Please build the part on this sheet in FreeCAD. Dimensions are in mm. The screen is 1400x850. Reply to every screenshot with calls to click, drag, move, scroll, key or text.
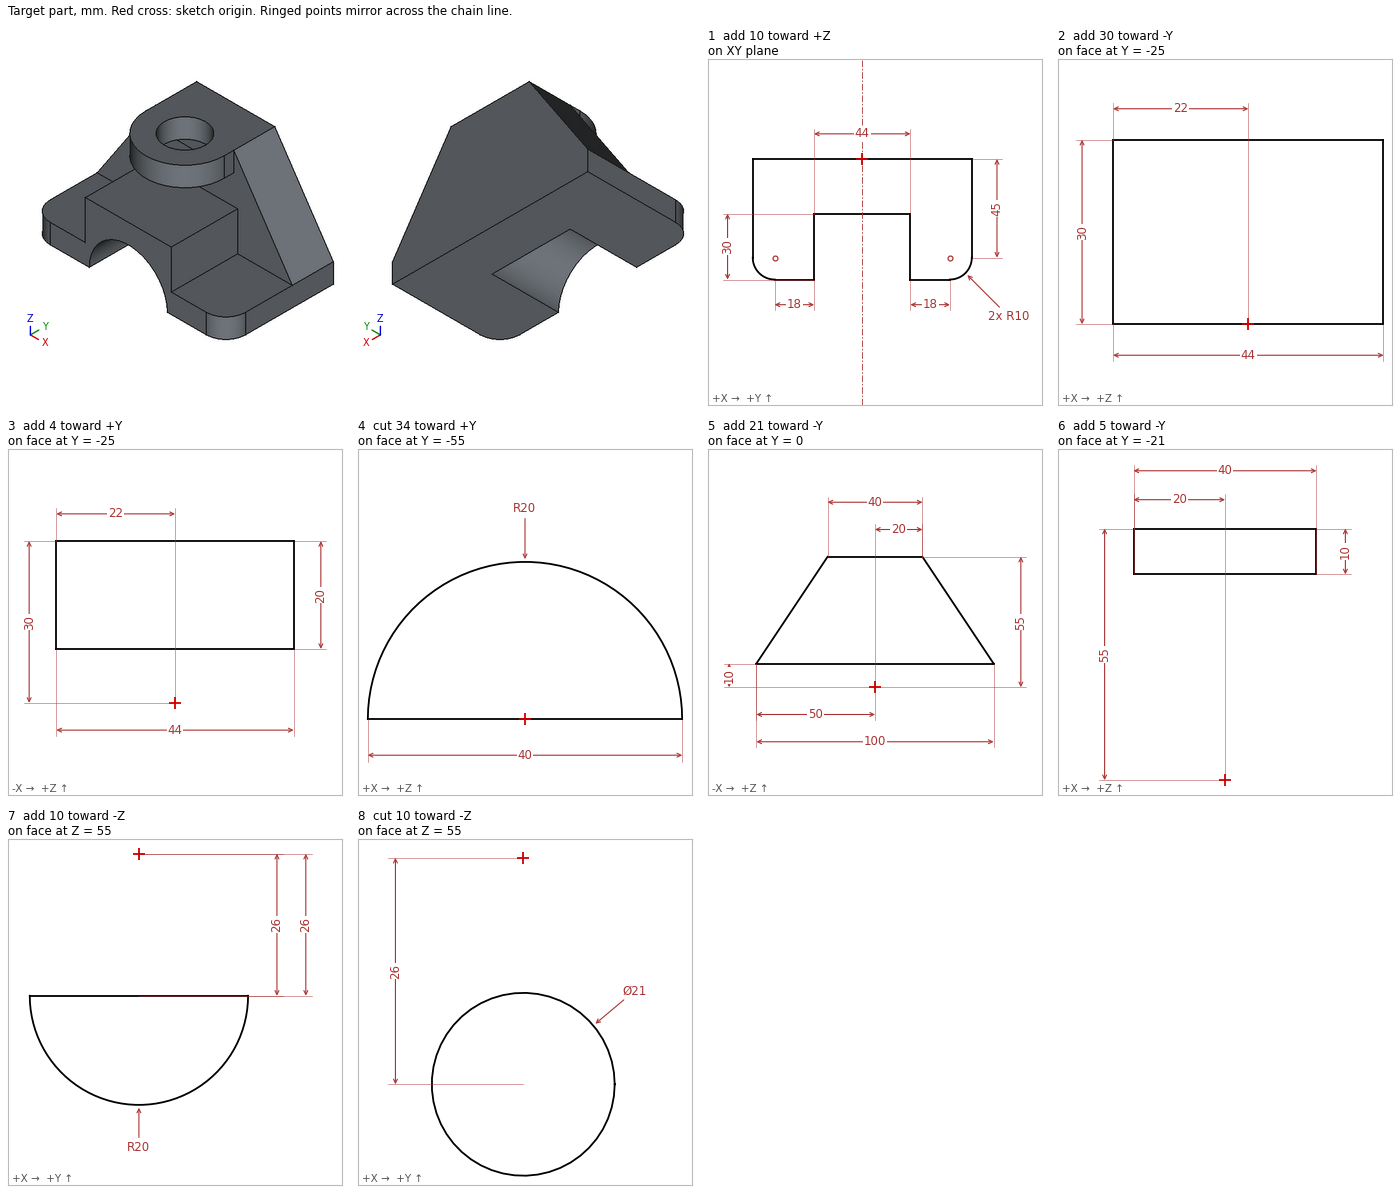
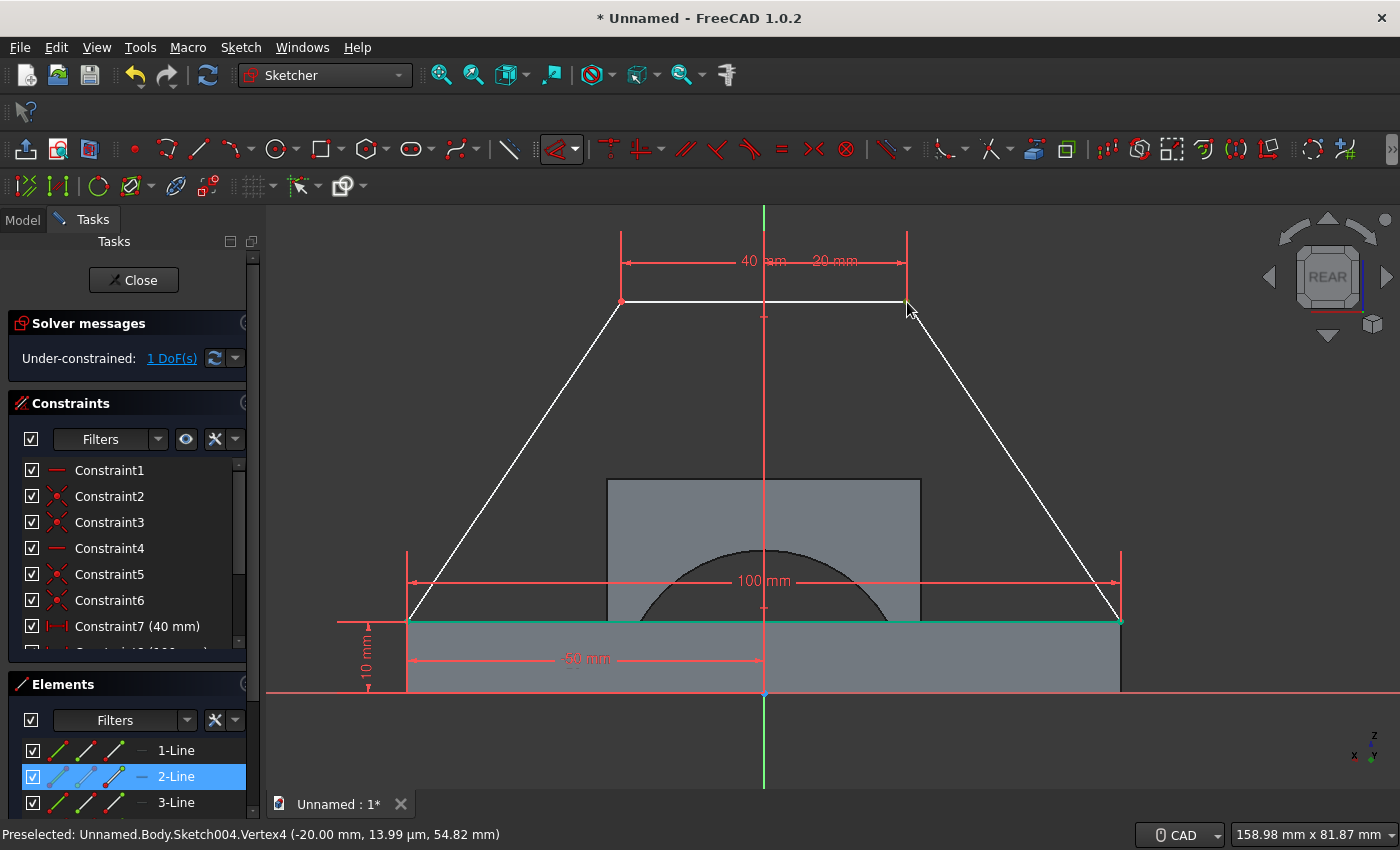
click(578, 150)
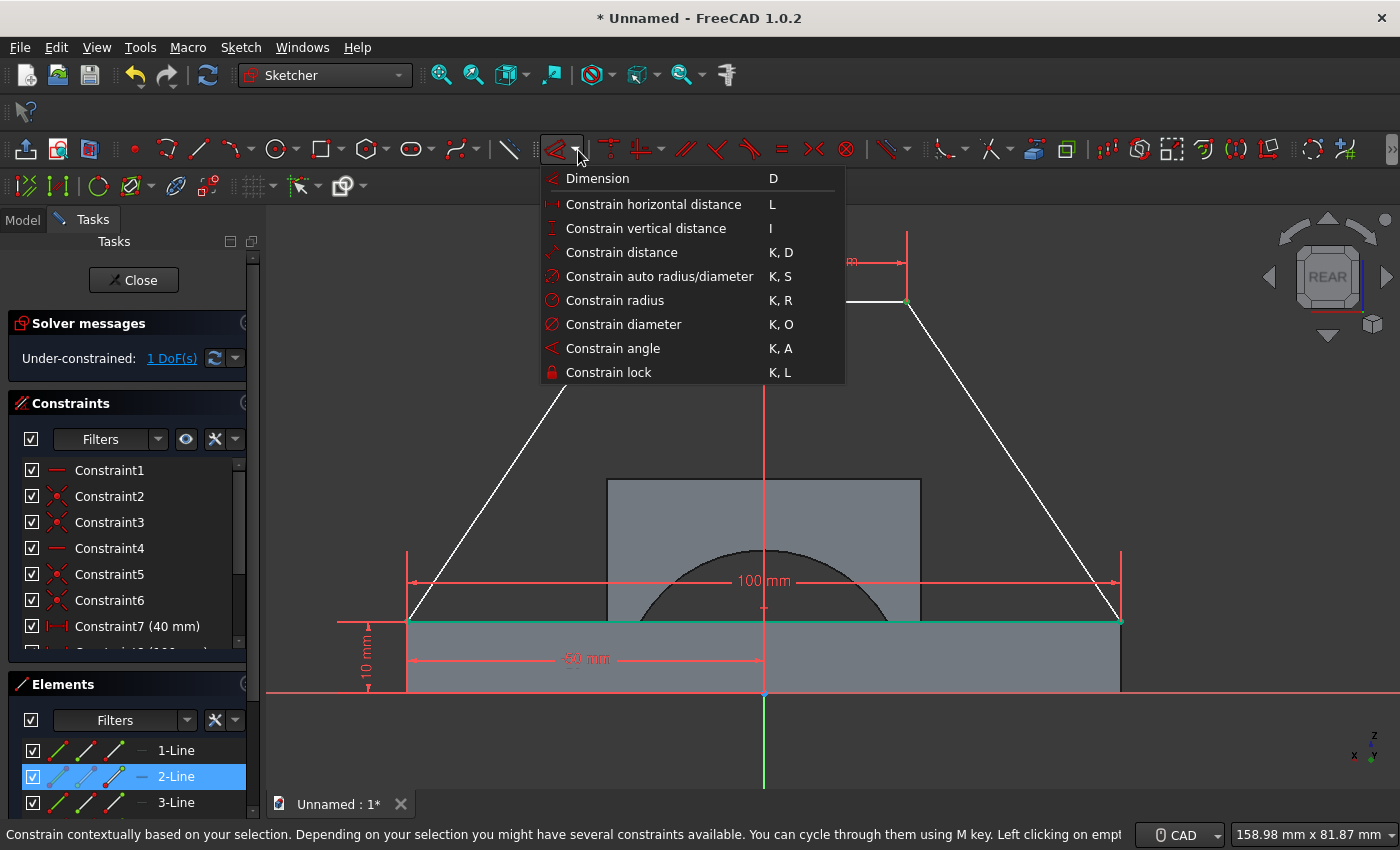
click(693, 228)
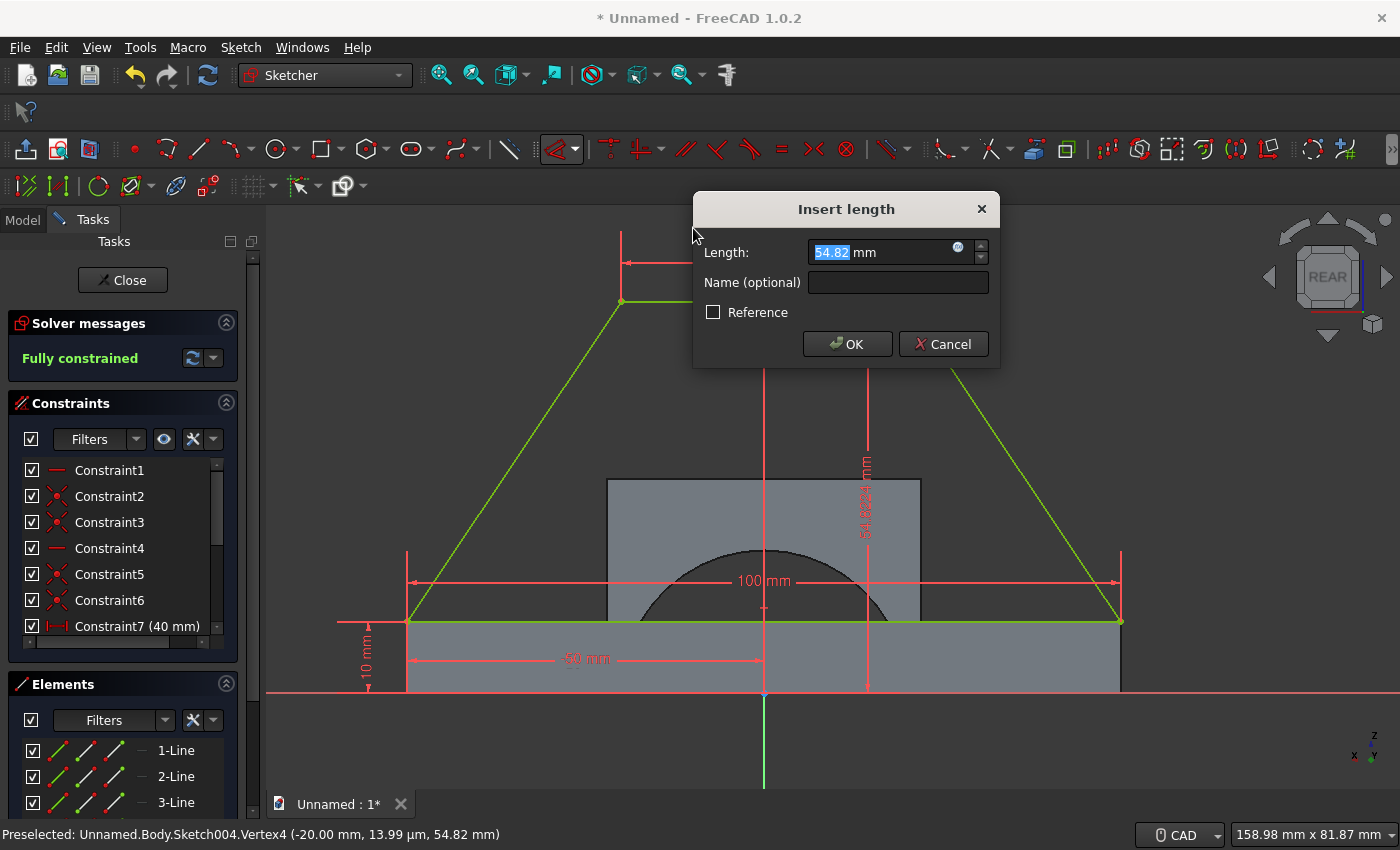
text(55)
key(Return)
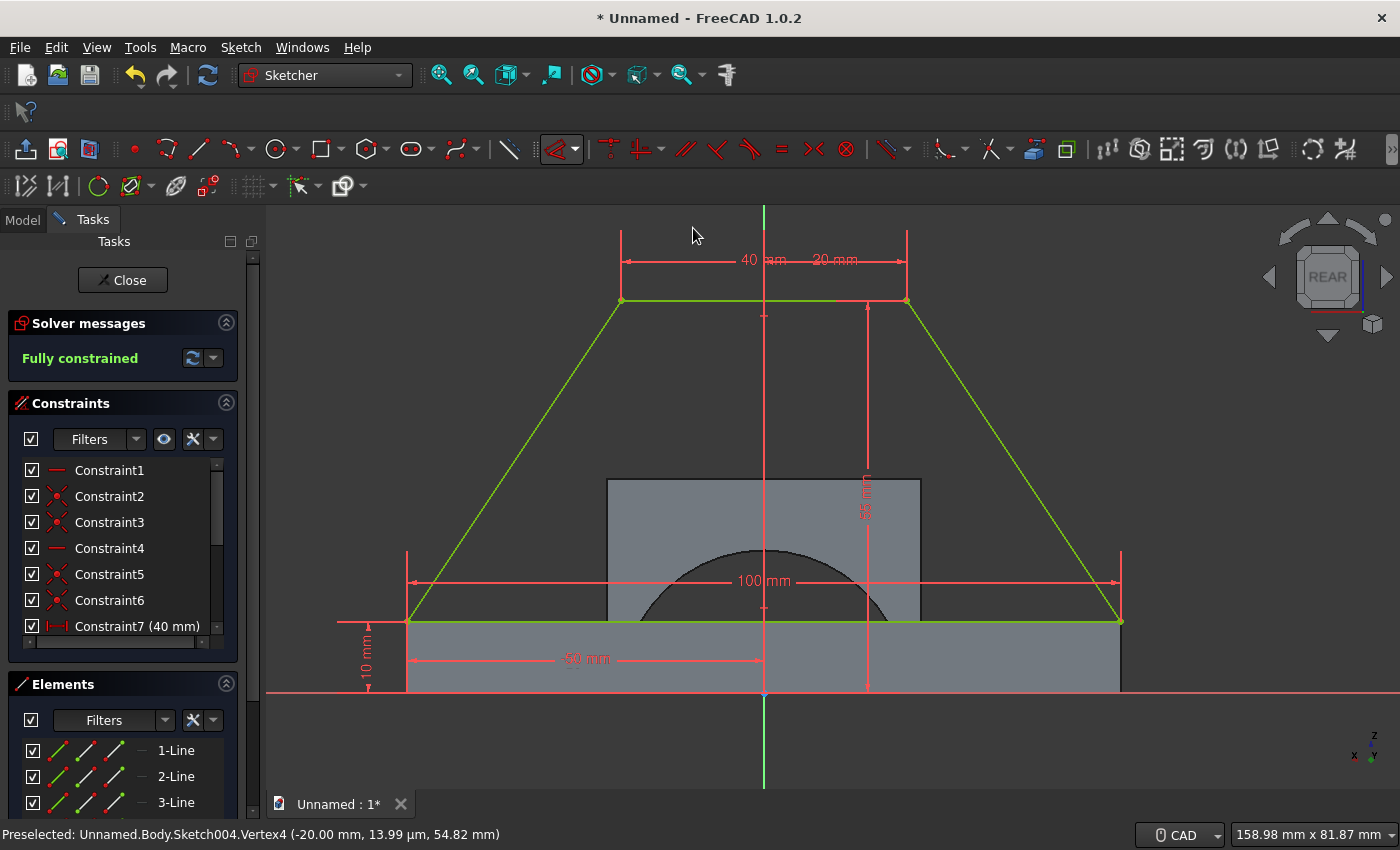
click(123, 280)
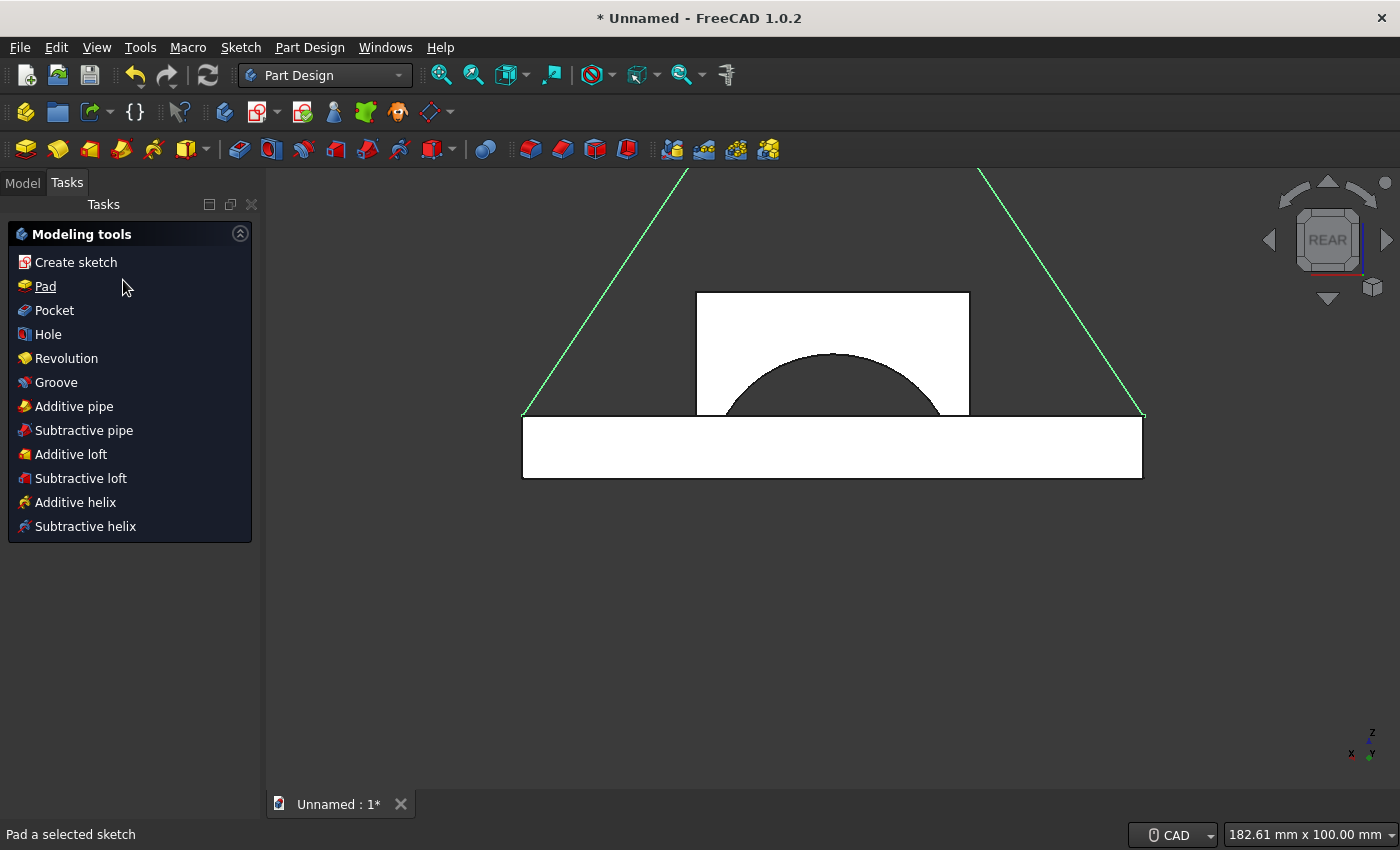
click(26, 150)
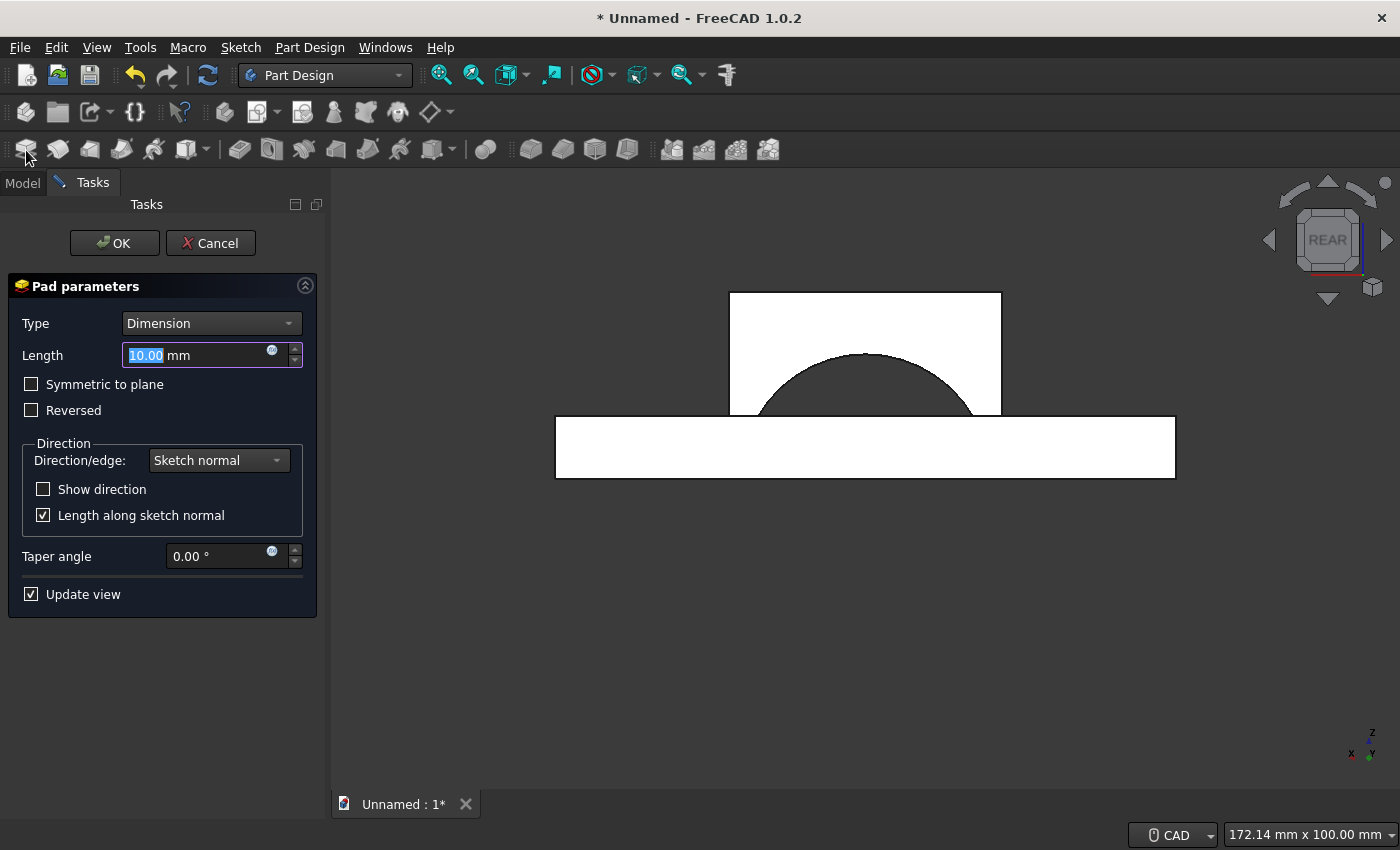
text(21)
key(Tab)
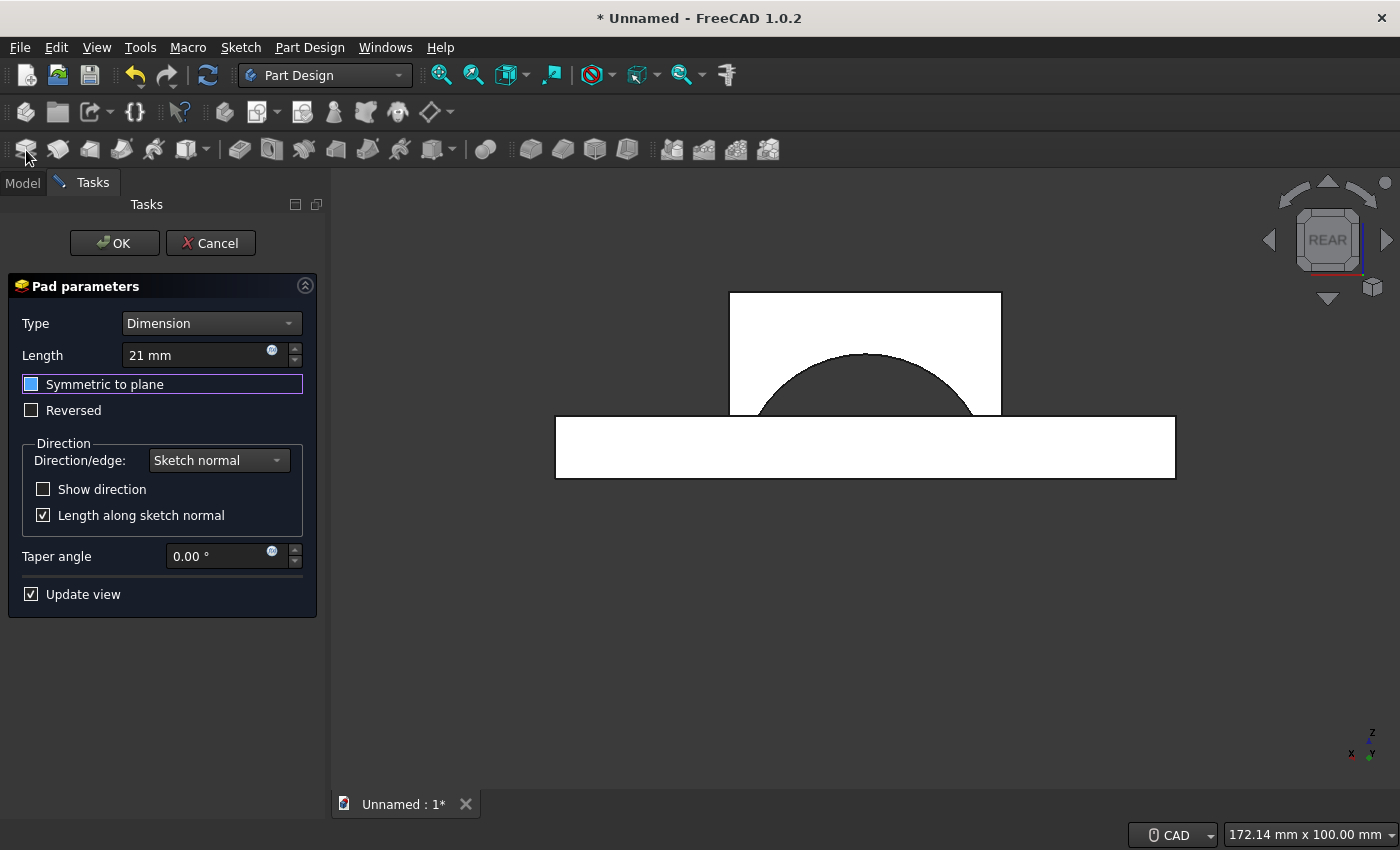
click(30, 410)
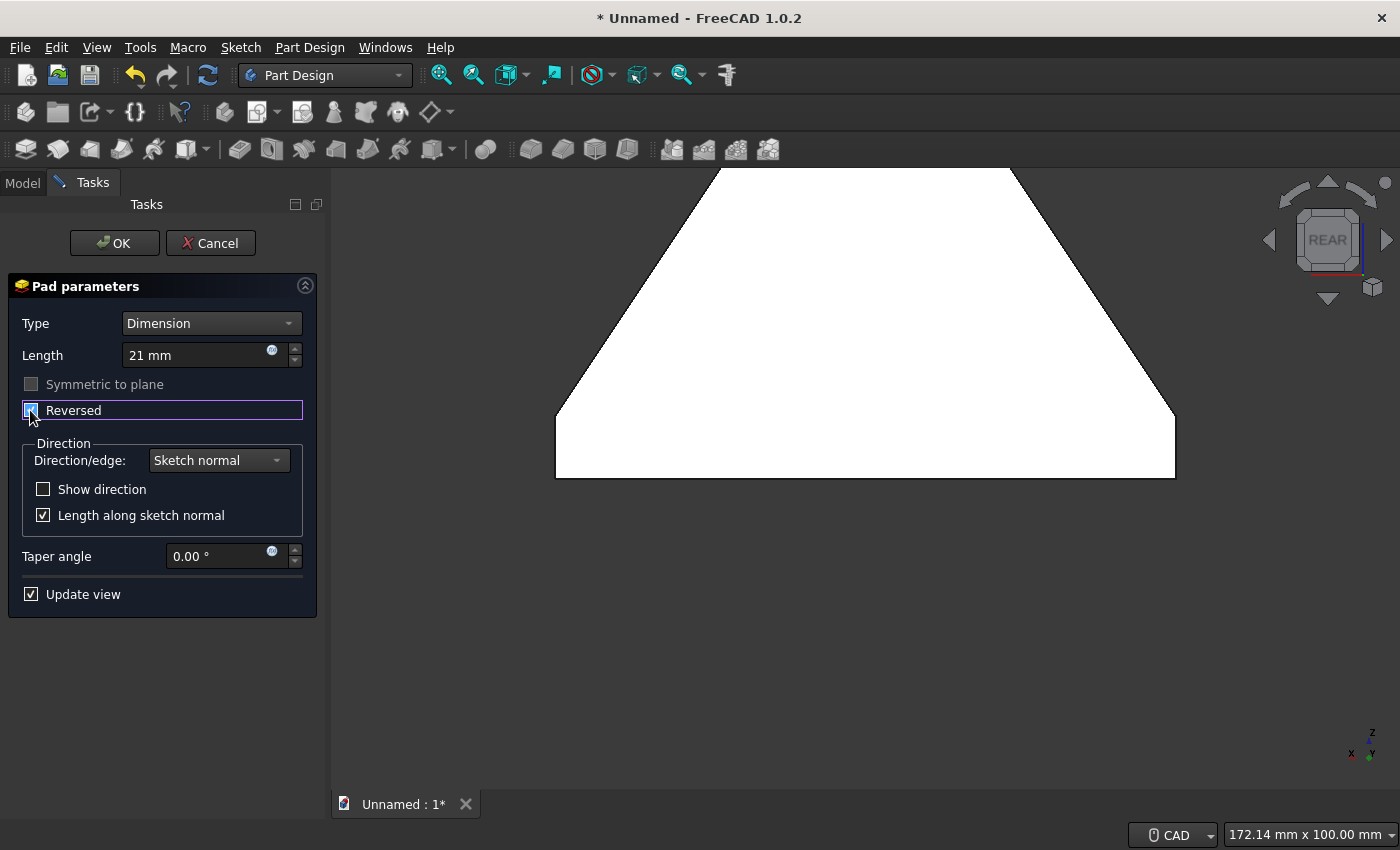
click(115, 243)